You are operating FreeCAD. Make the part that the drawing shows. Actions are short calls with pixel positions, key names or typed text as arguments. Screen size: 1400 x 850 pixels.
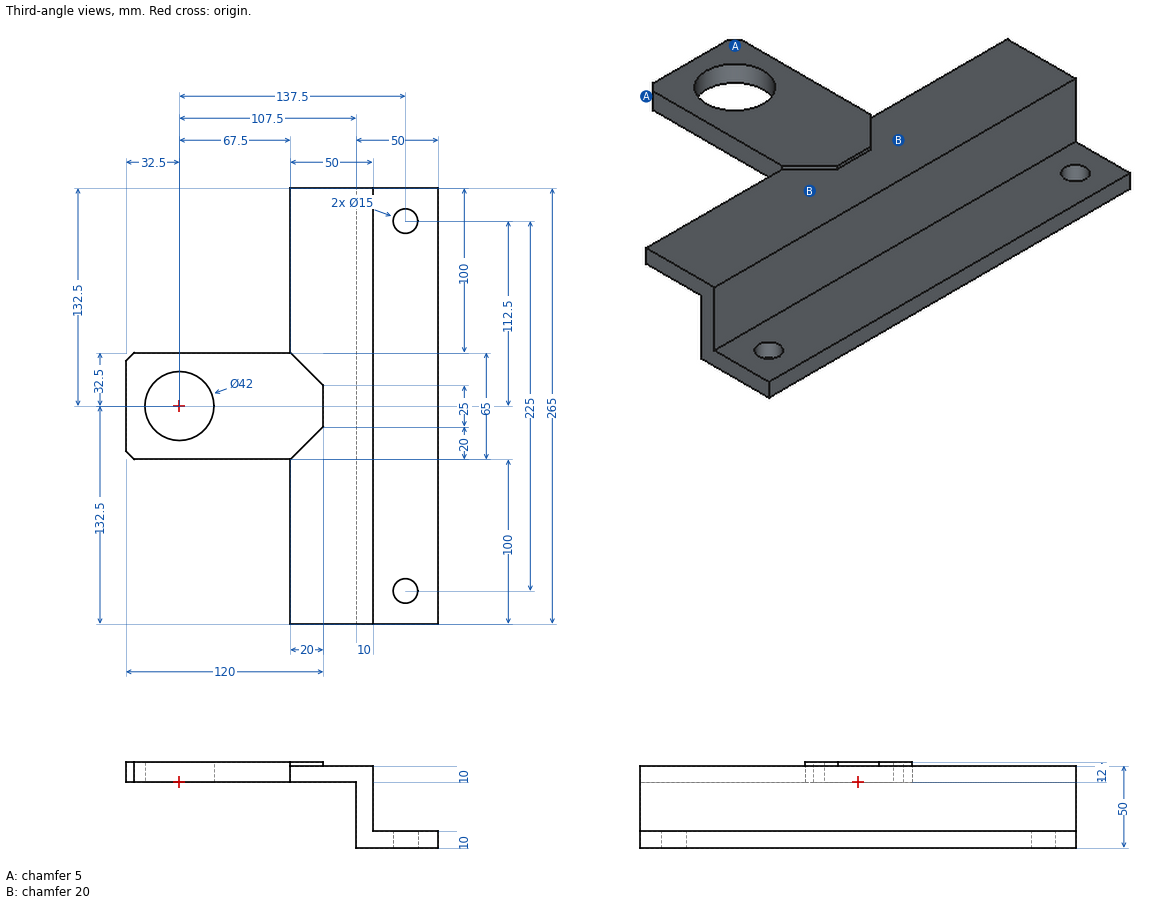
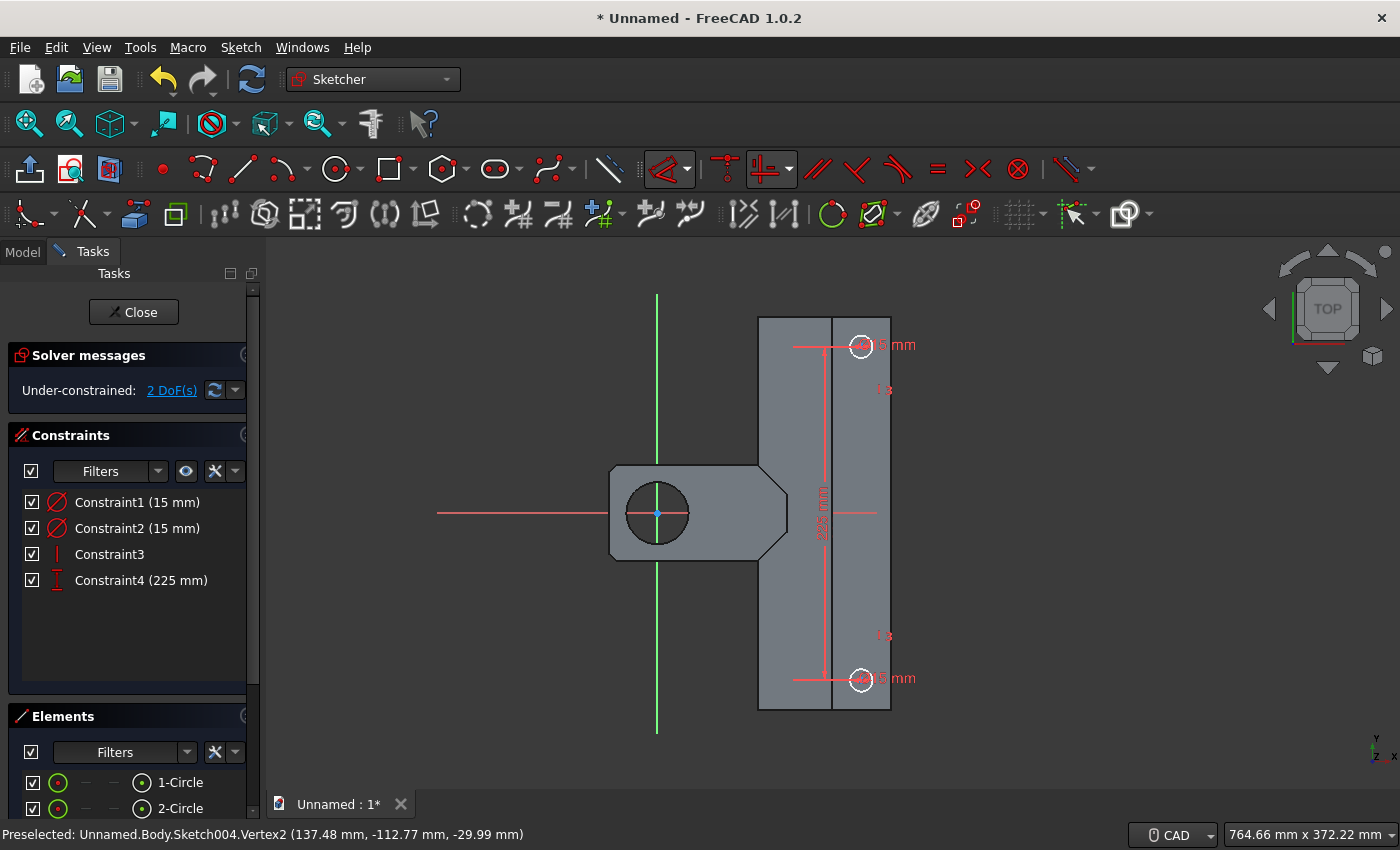
click(861, 347)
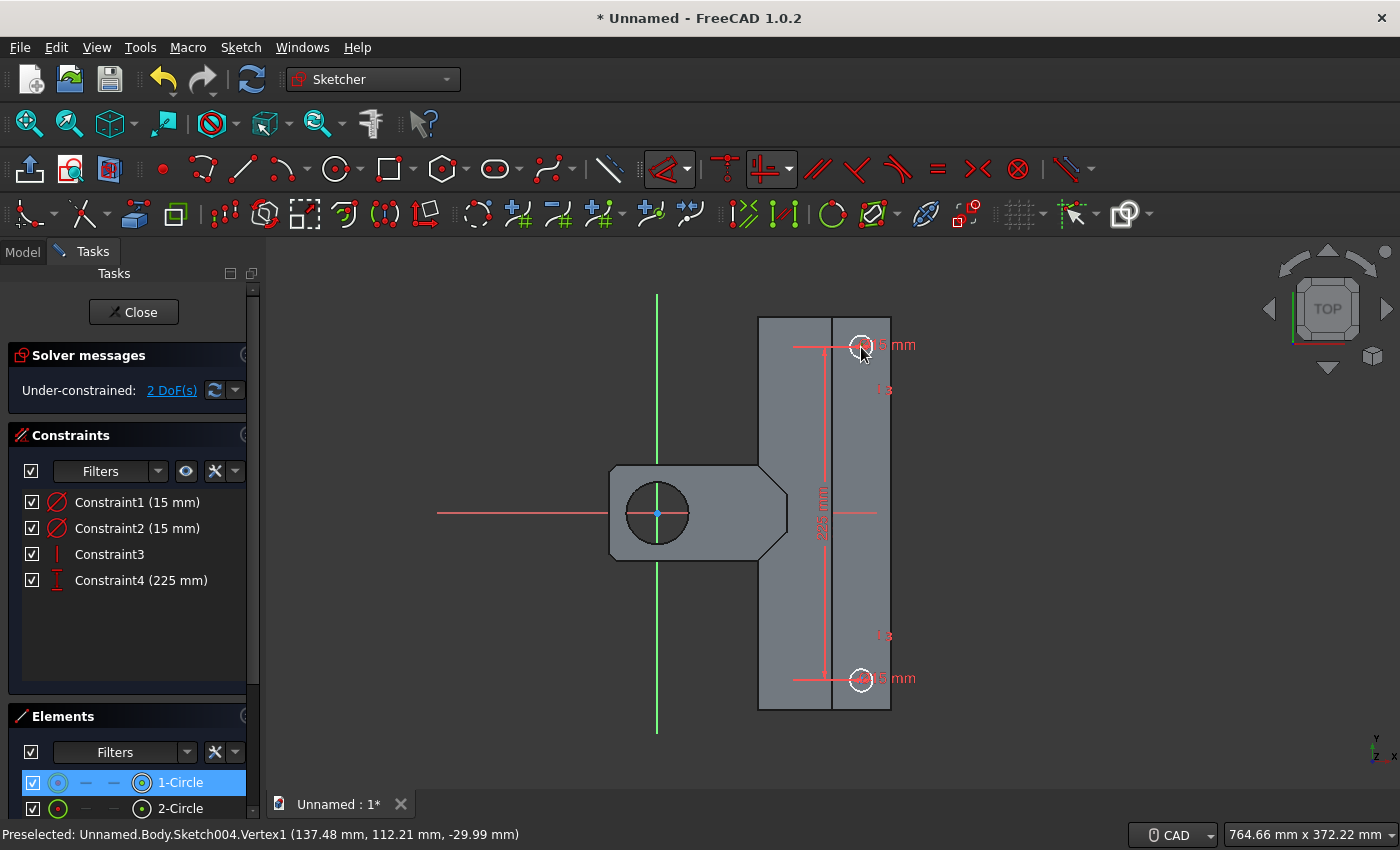
click(690, 170)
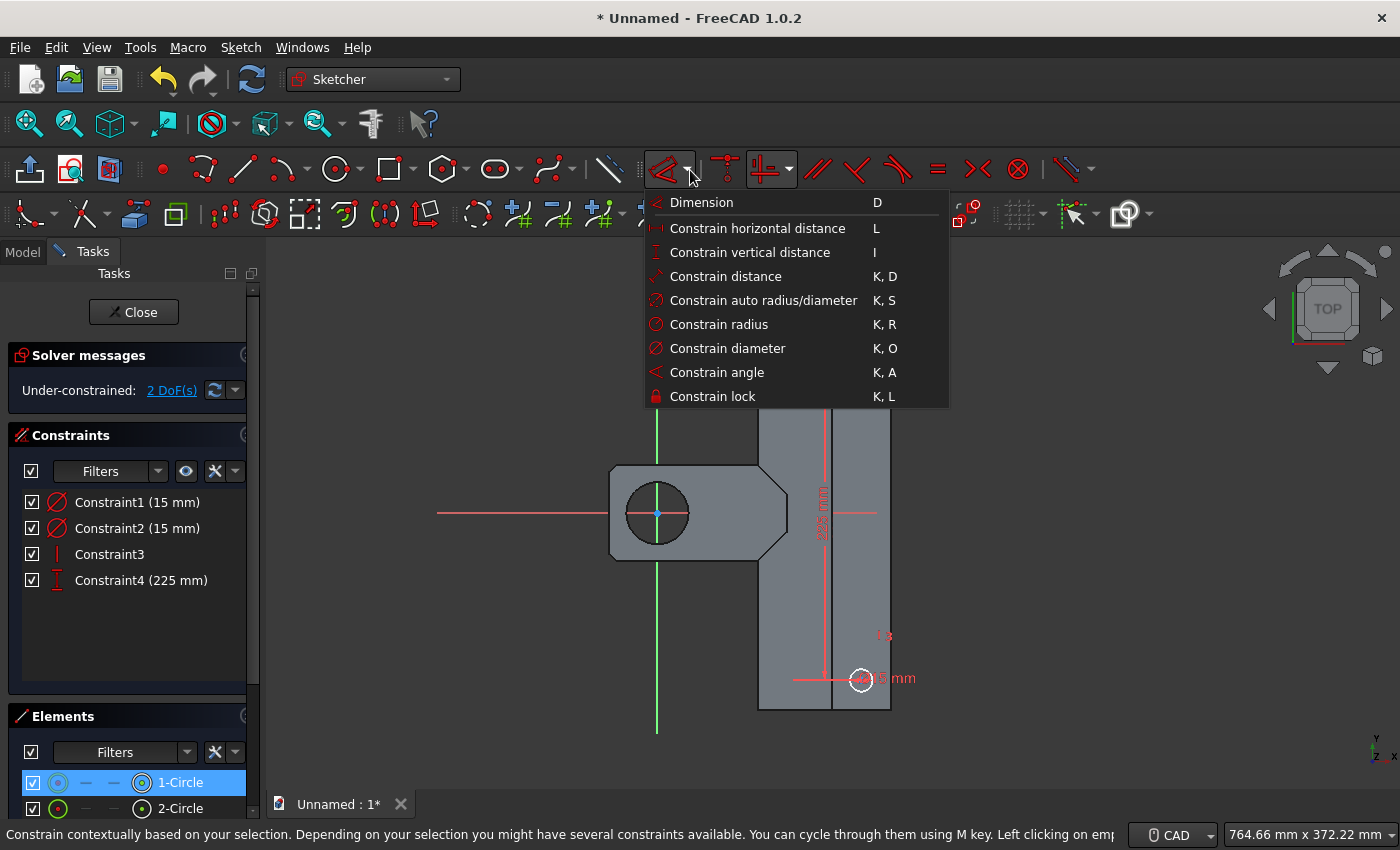
click(797, 228)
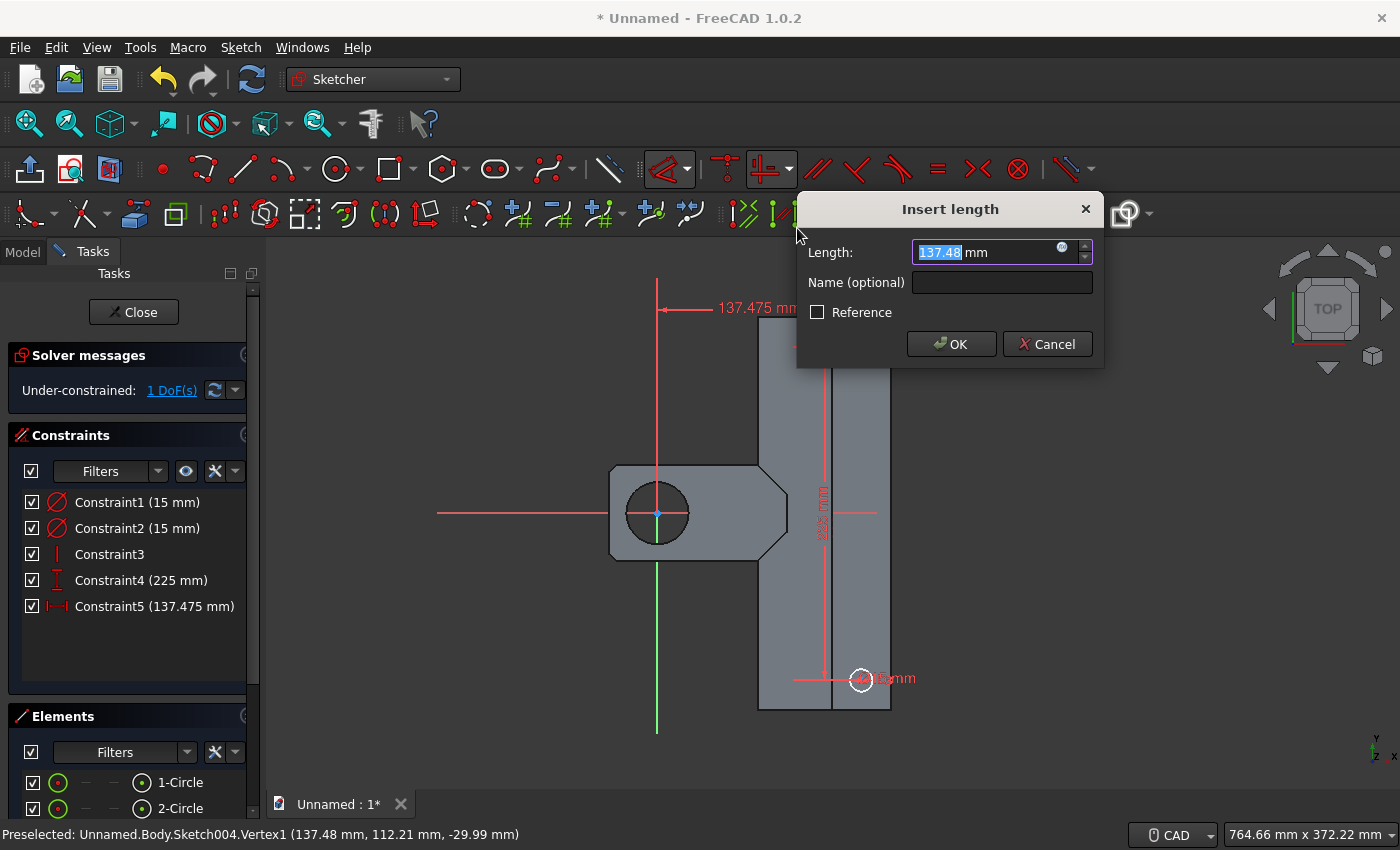
text(137.5)
key(Return)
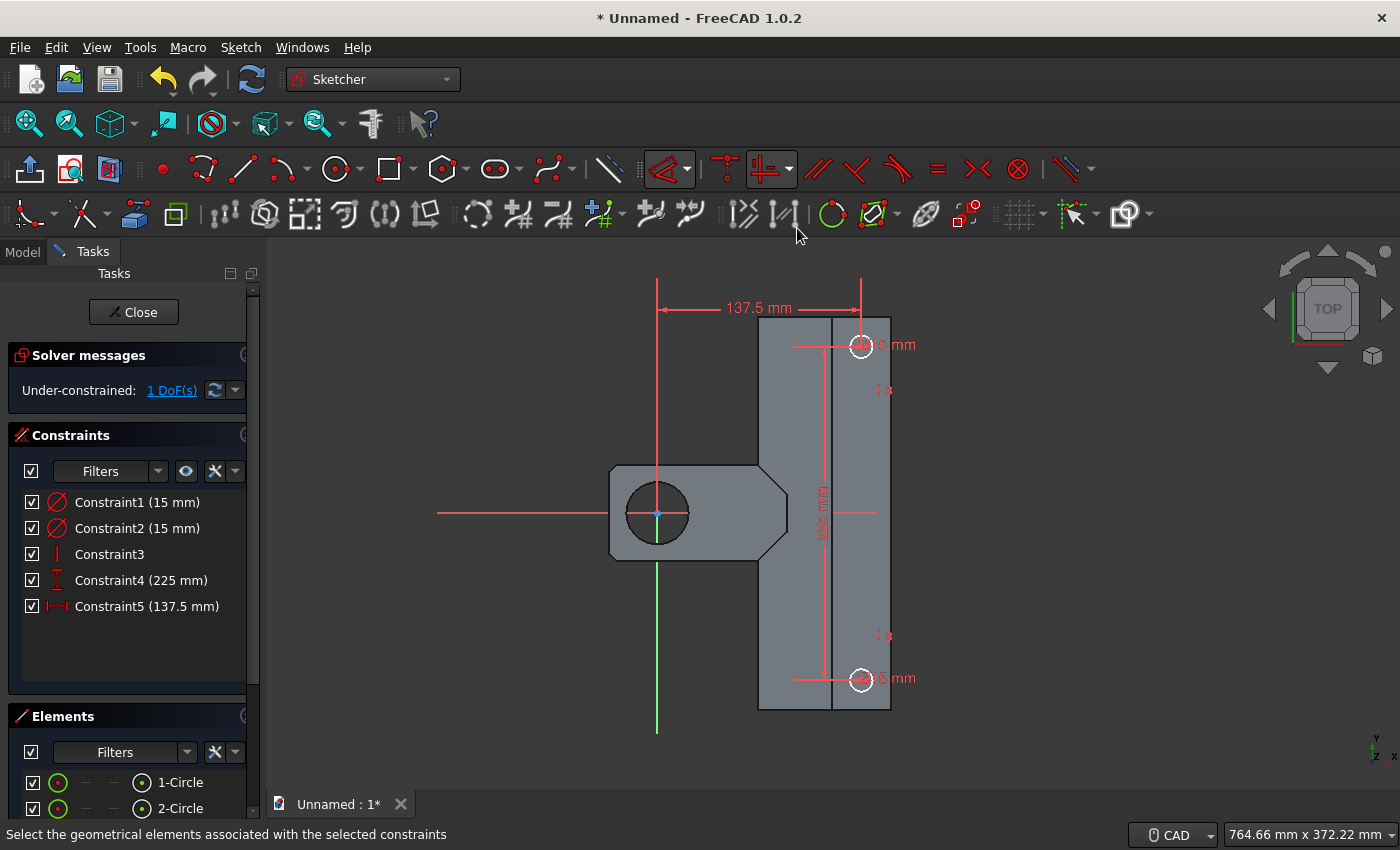
click(861, 347)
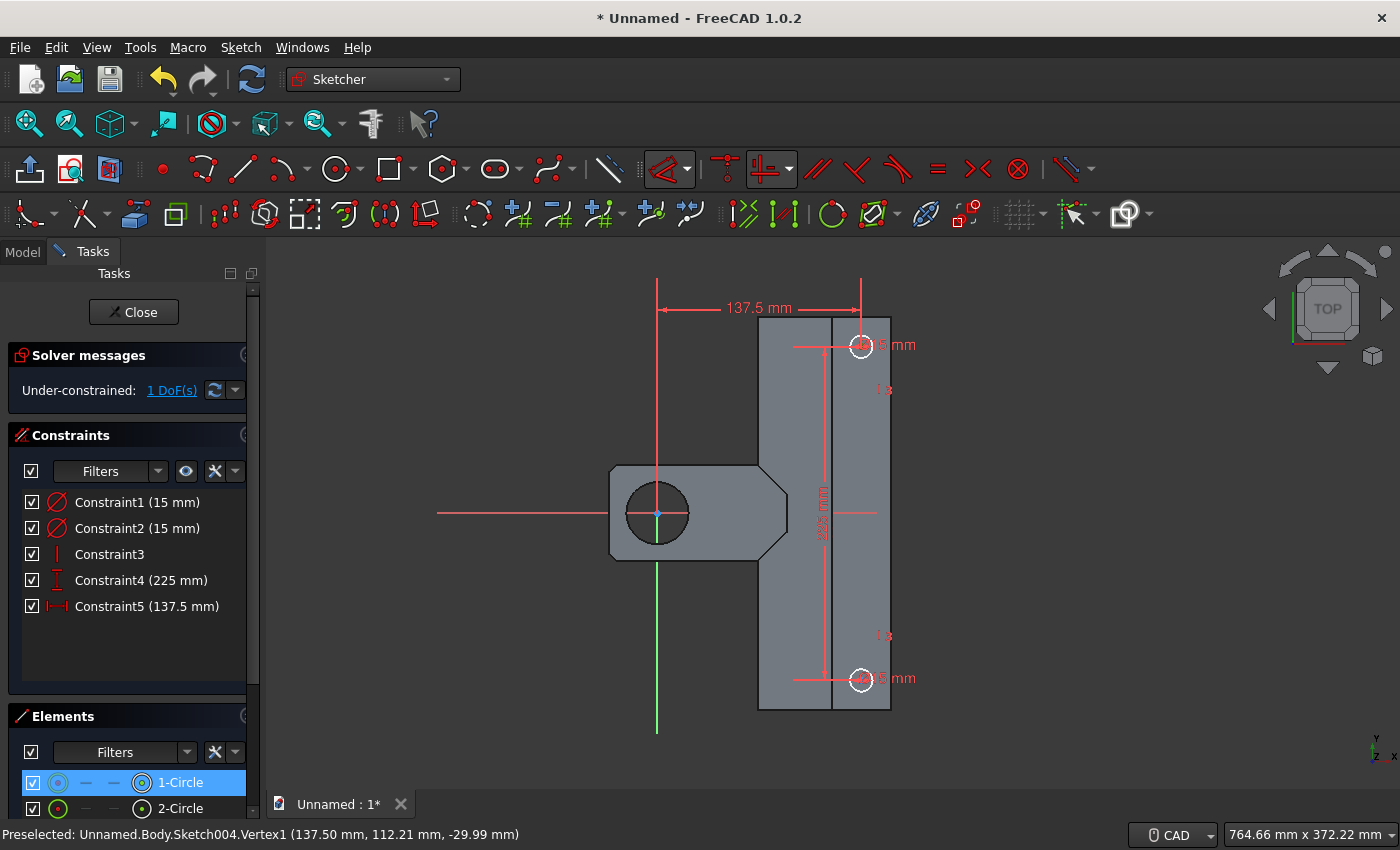
key(i)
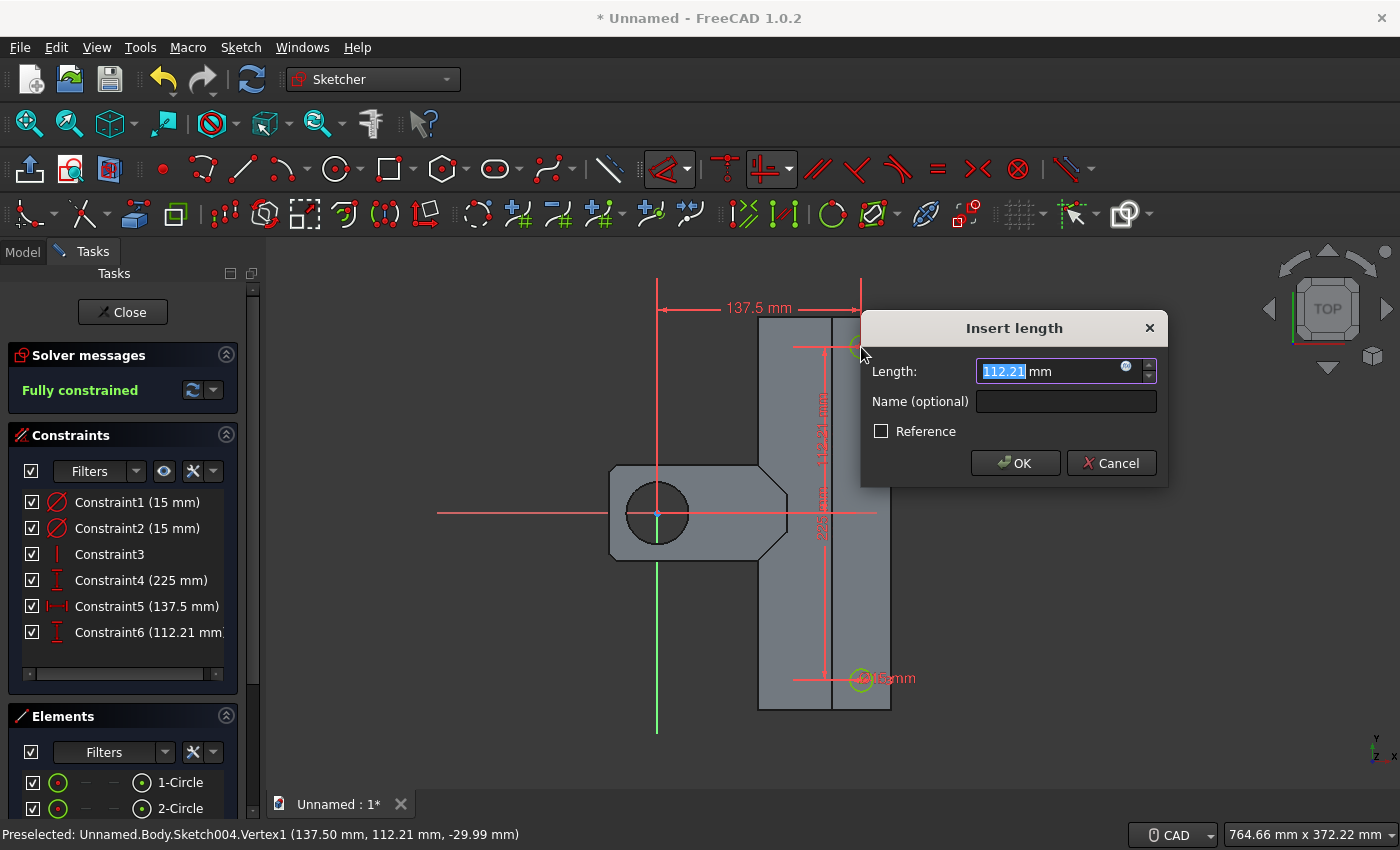
text(112.5)
key(Return)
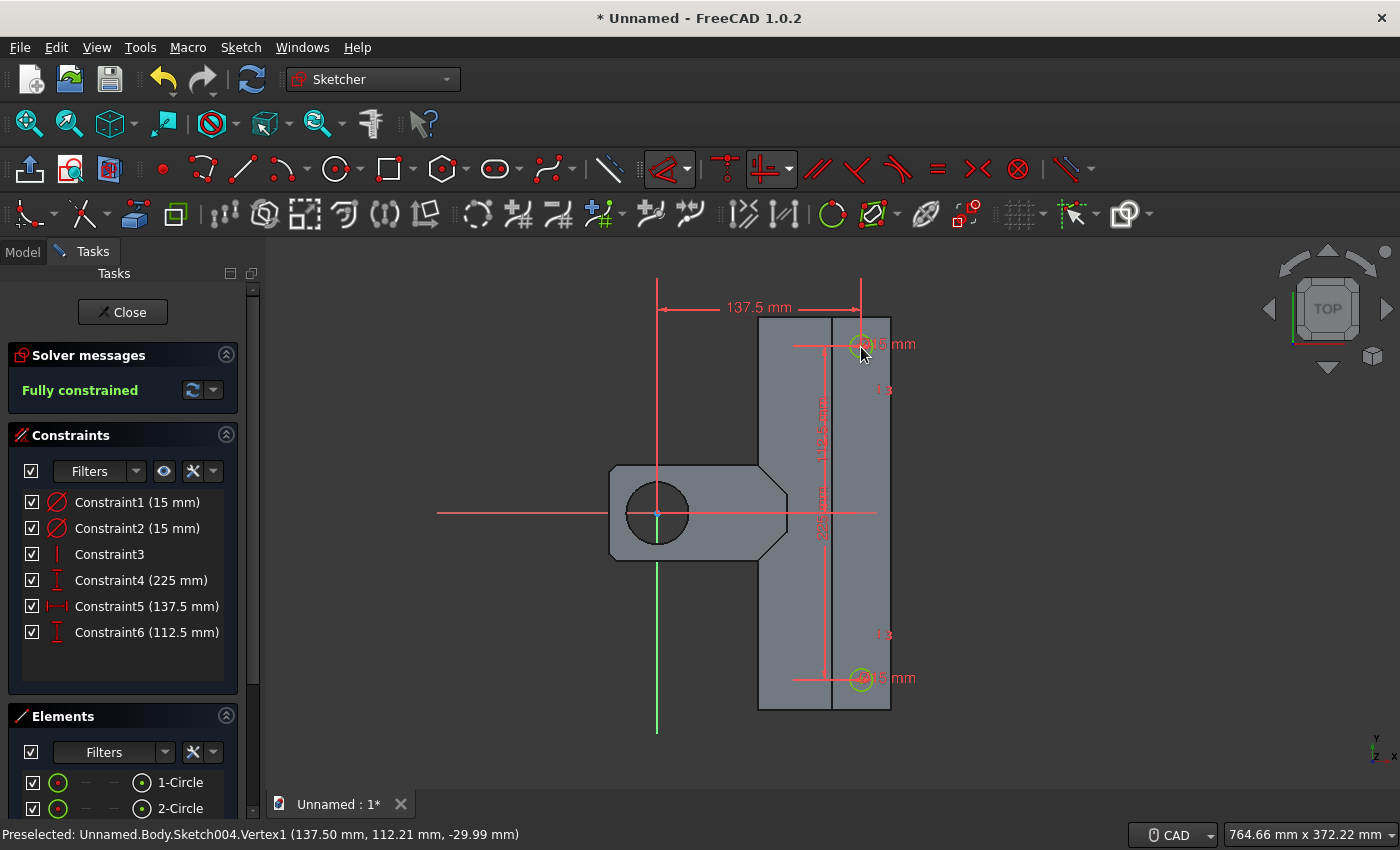
click(123, 312)